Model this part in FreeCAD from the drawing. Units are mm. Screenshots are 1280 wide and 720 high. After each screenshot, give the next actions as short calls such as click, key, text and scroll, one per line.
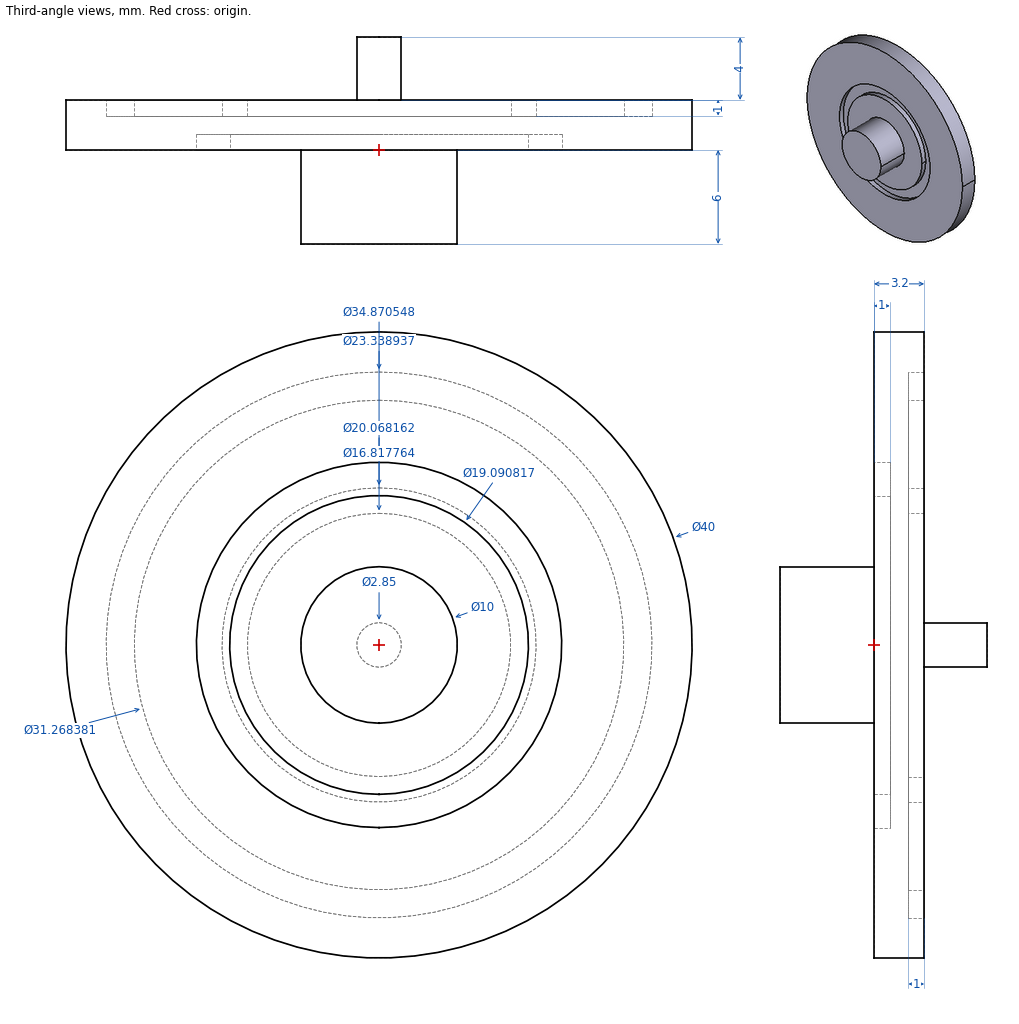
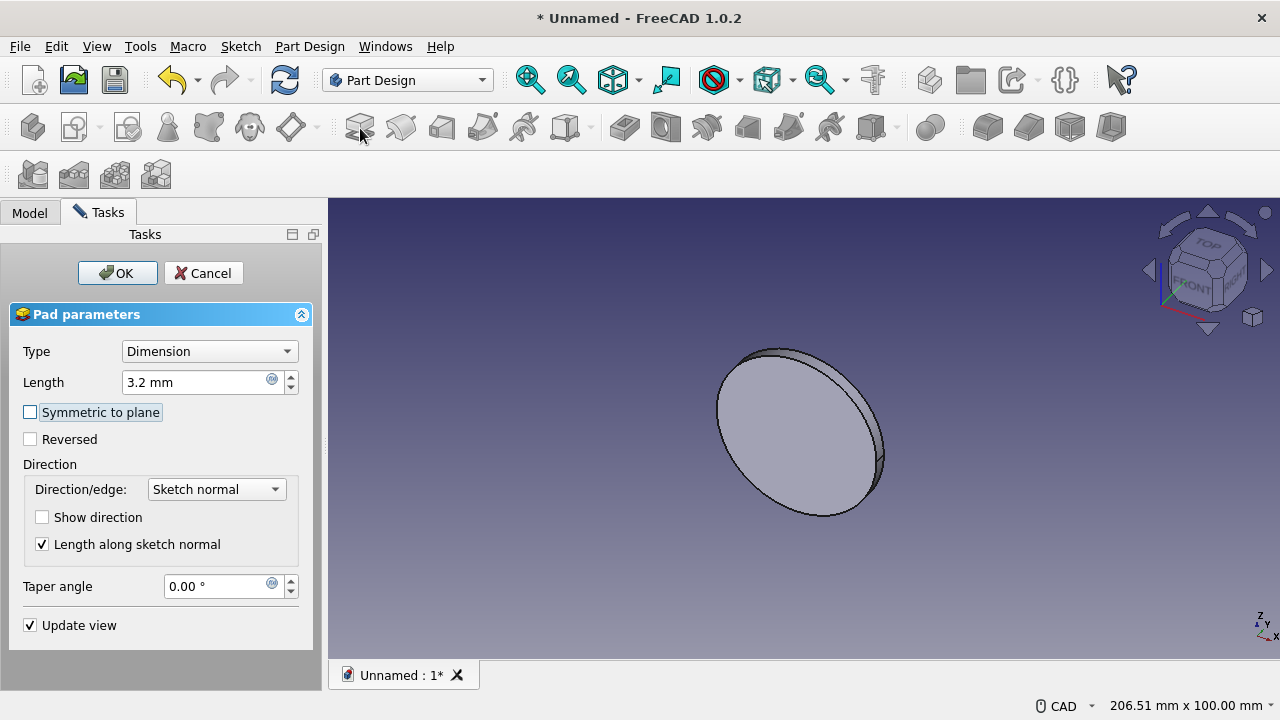
click(31, 439)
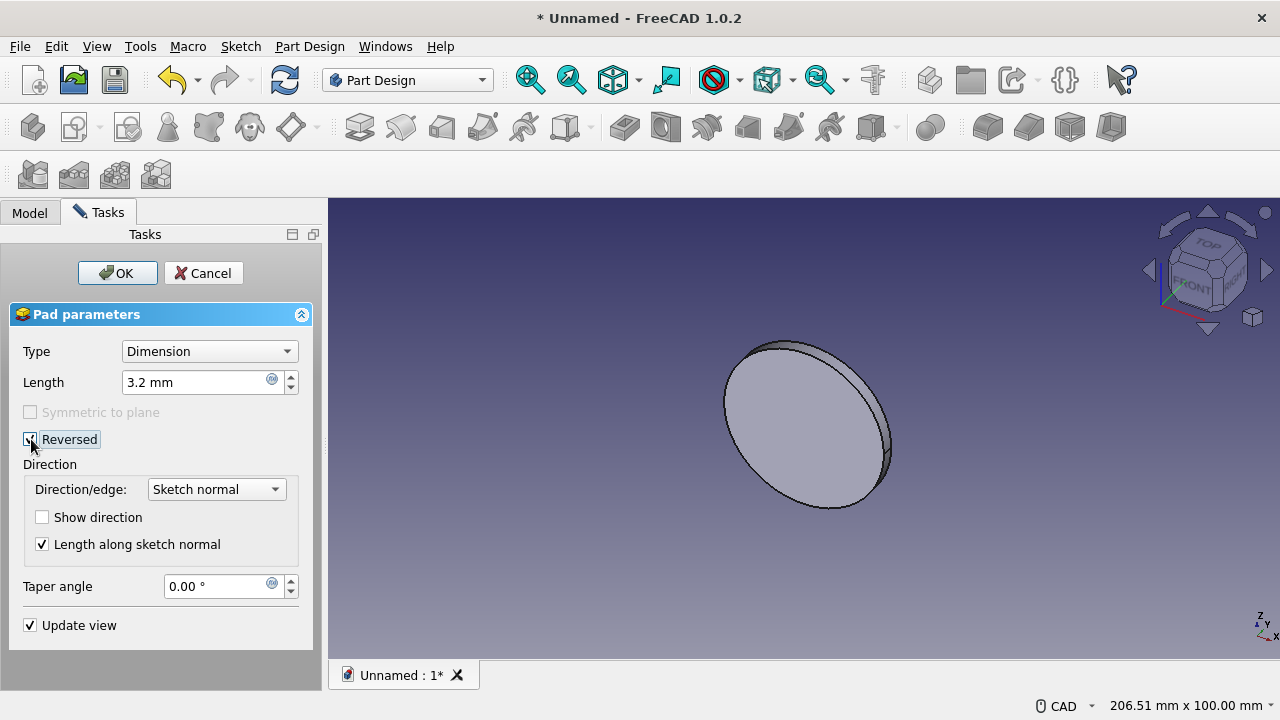
click(118, 273)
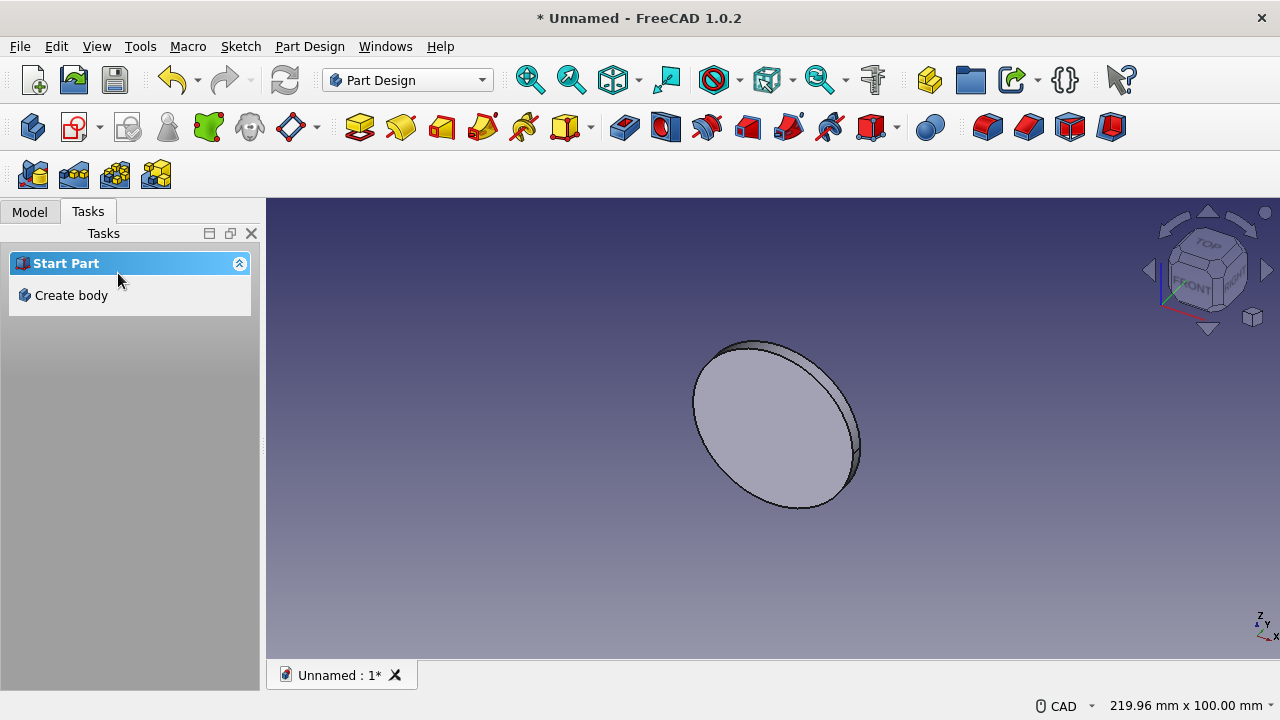
click(773, 427)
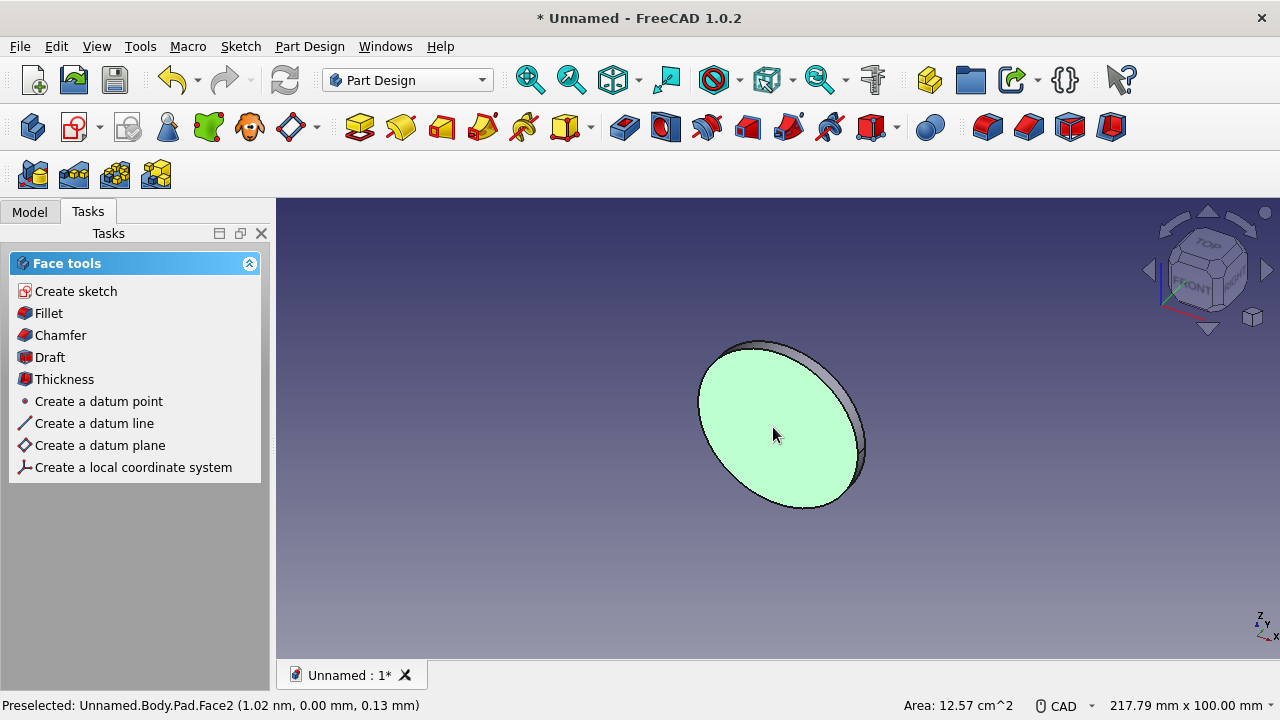
click(74, 128)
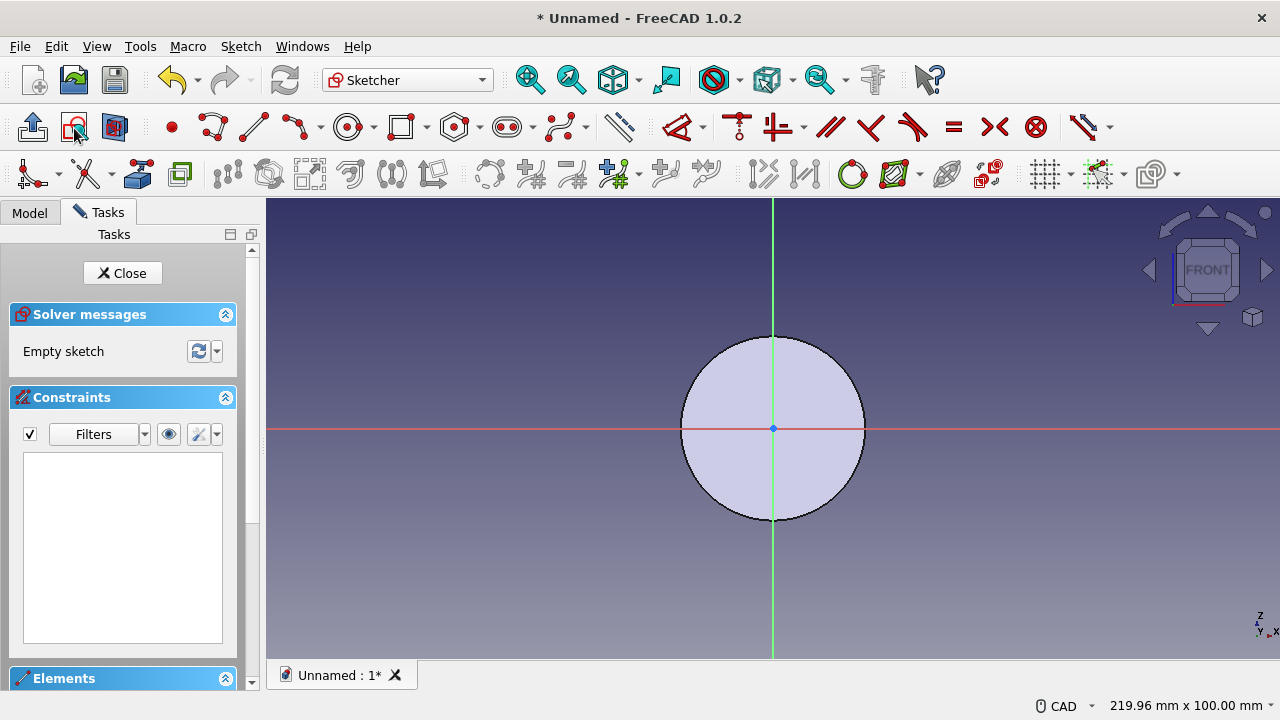
scroll(787, 428, up, 9)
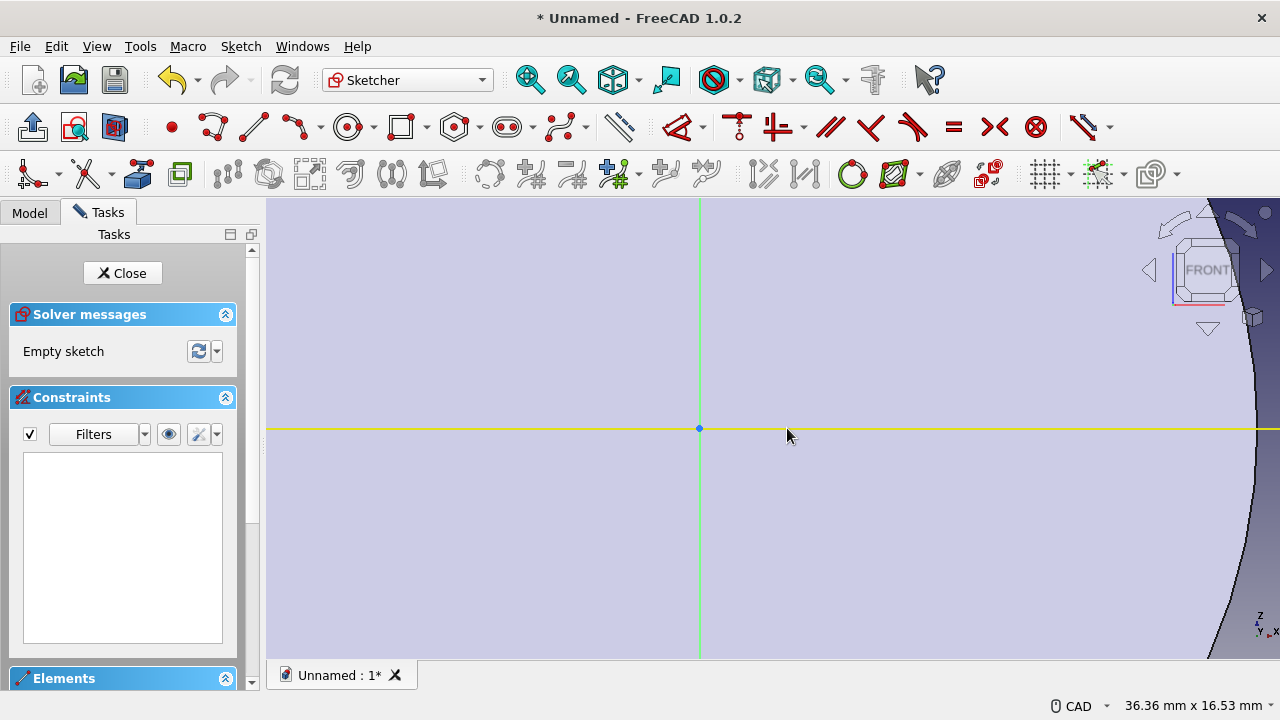
click(348, 128)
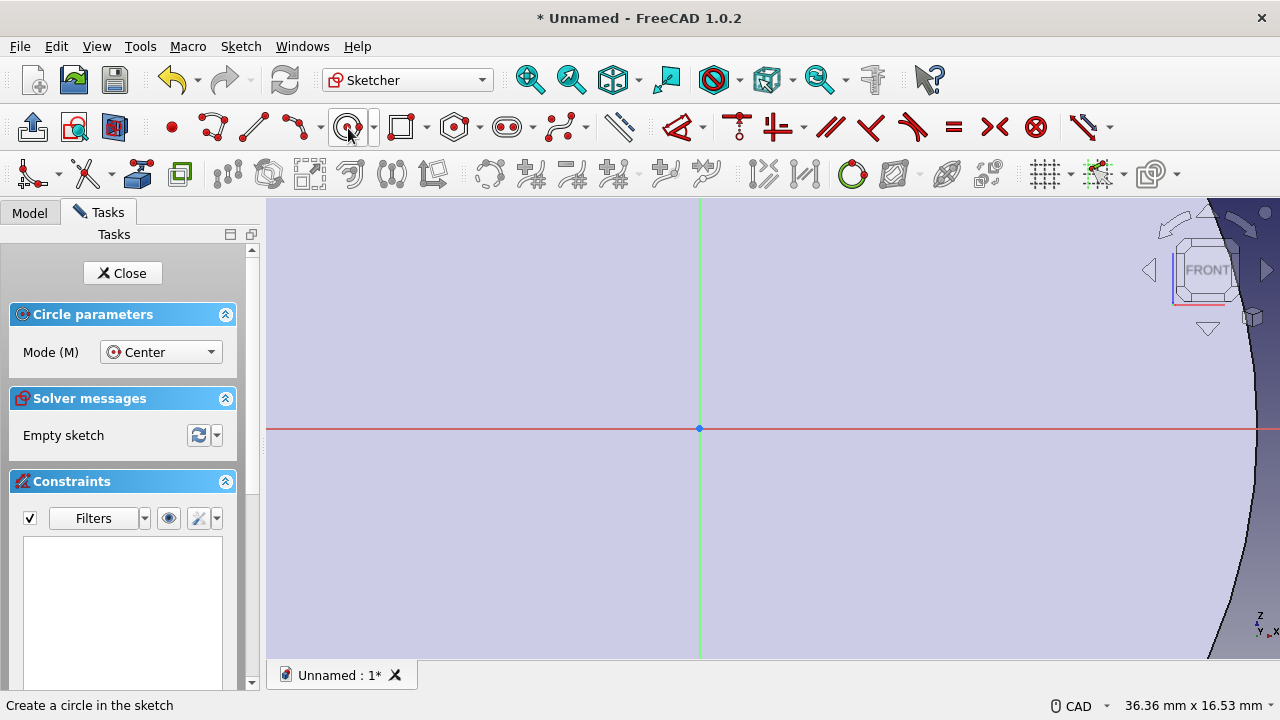
click(700, 428)
move(798, 330)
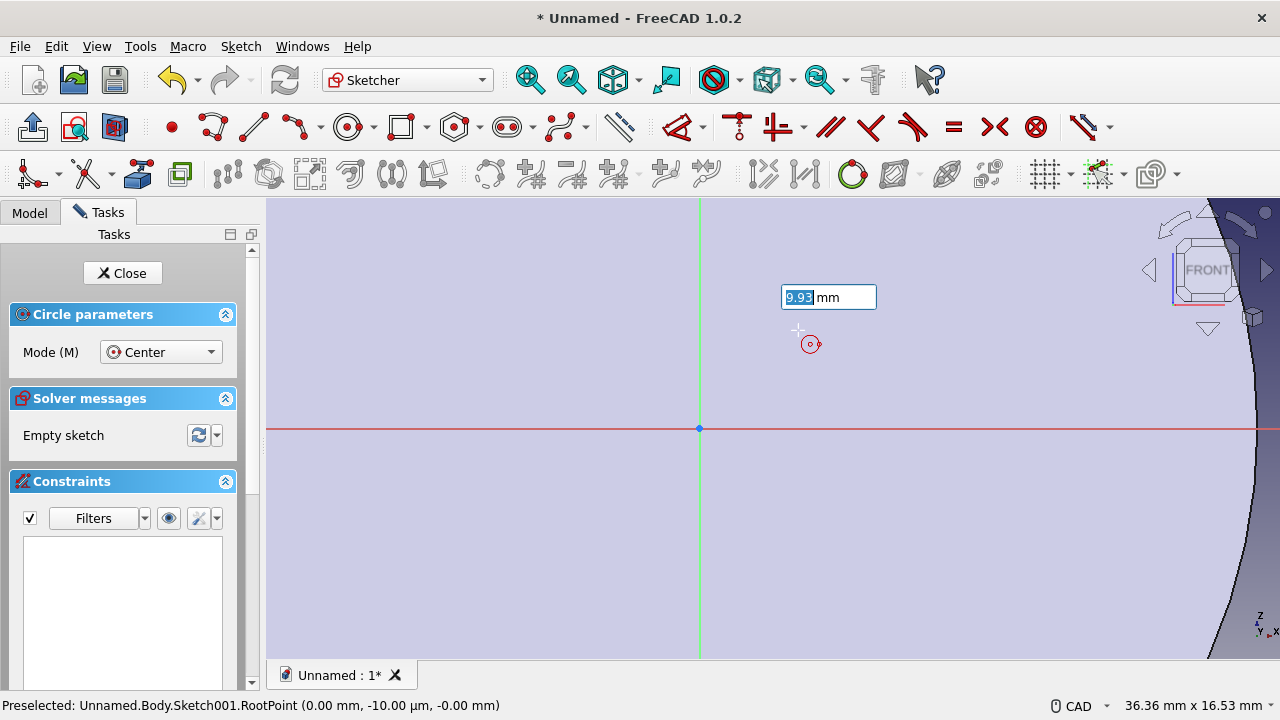
text(10)
key(Return)
key(Escape)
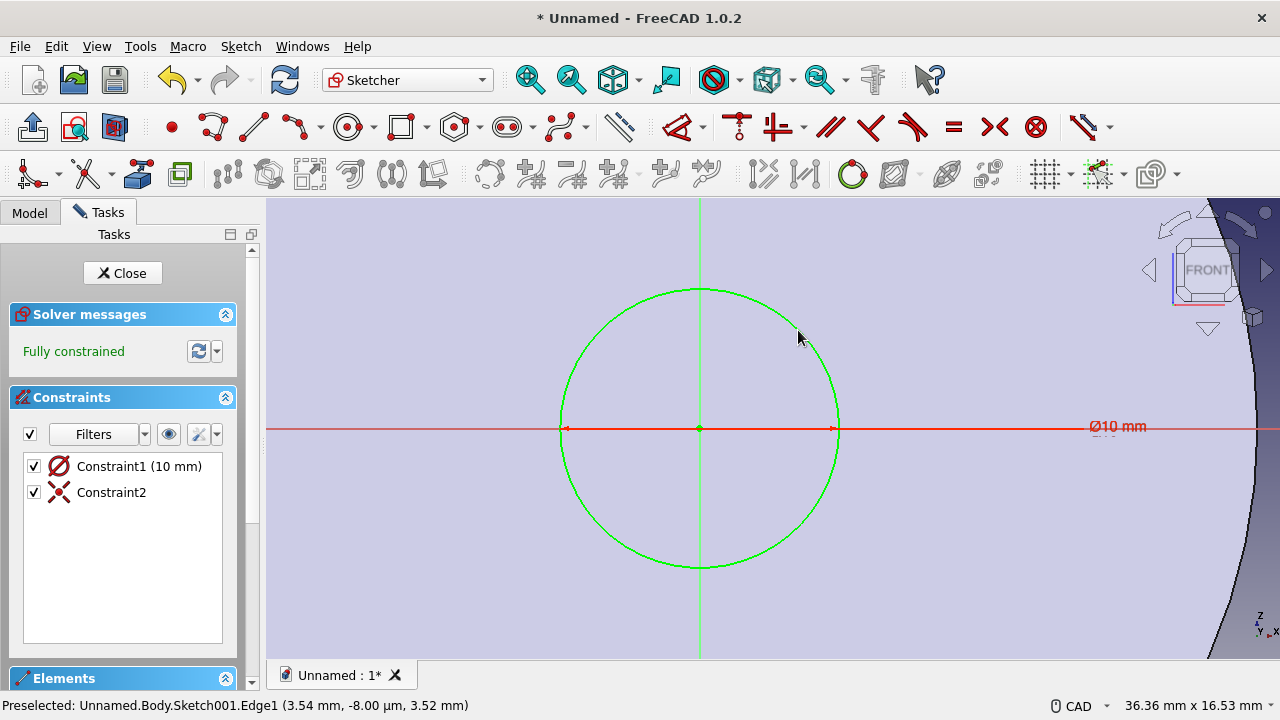
click(123, 273)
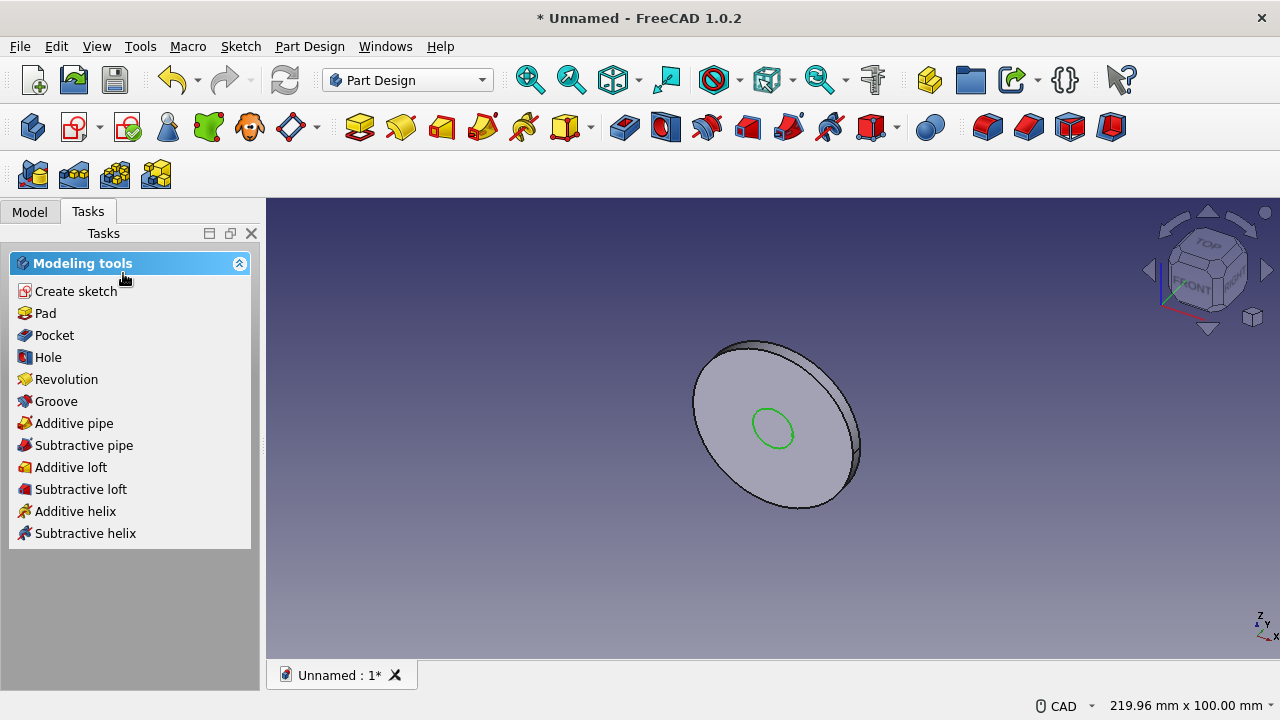
click(360, 128)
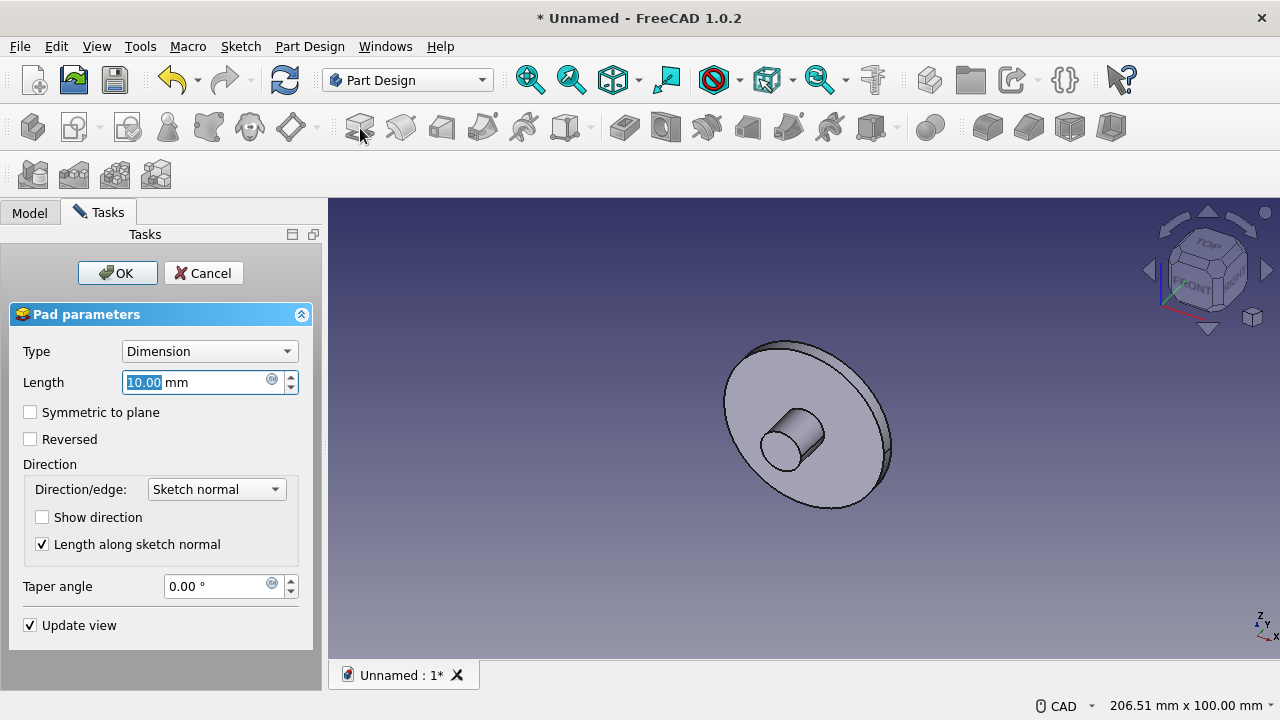
text(6)
key(Tab)